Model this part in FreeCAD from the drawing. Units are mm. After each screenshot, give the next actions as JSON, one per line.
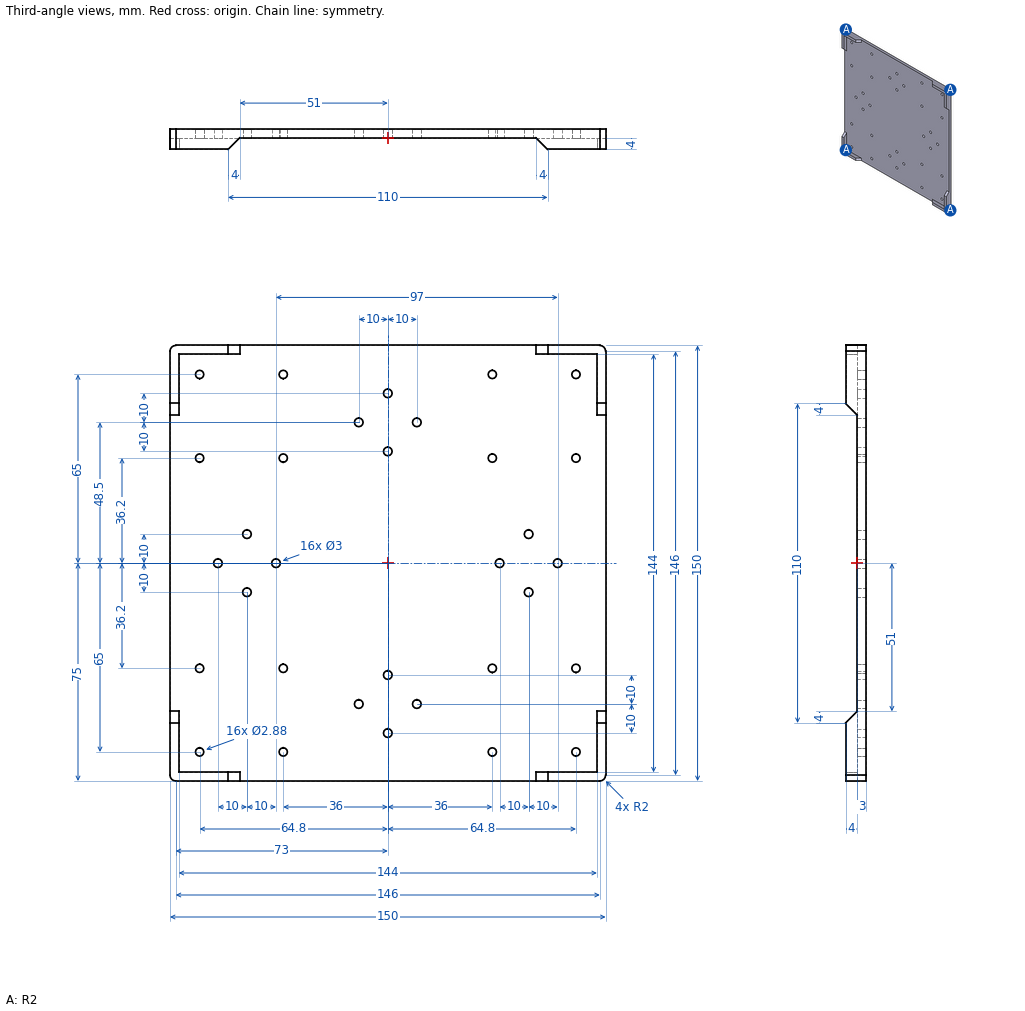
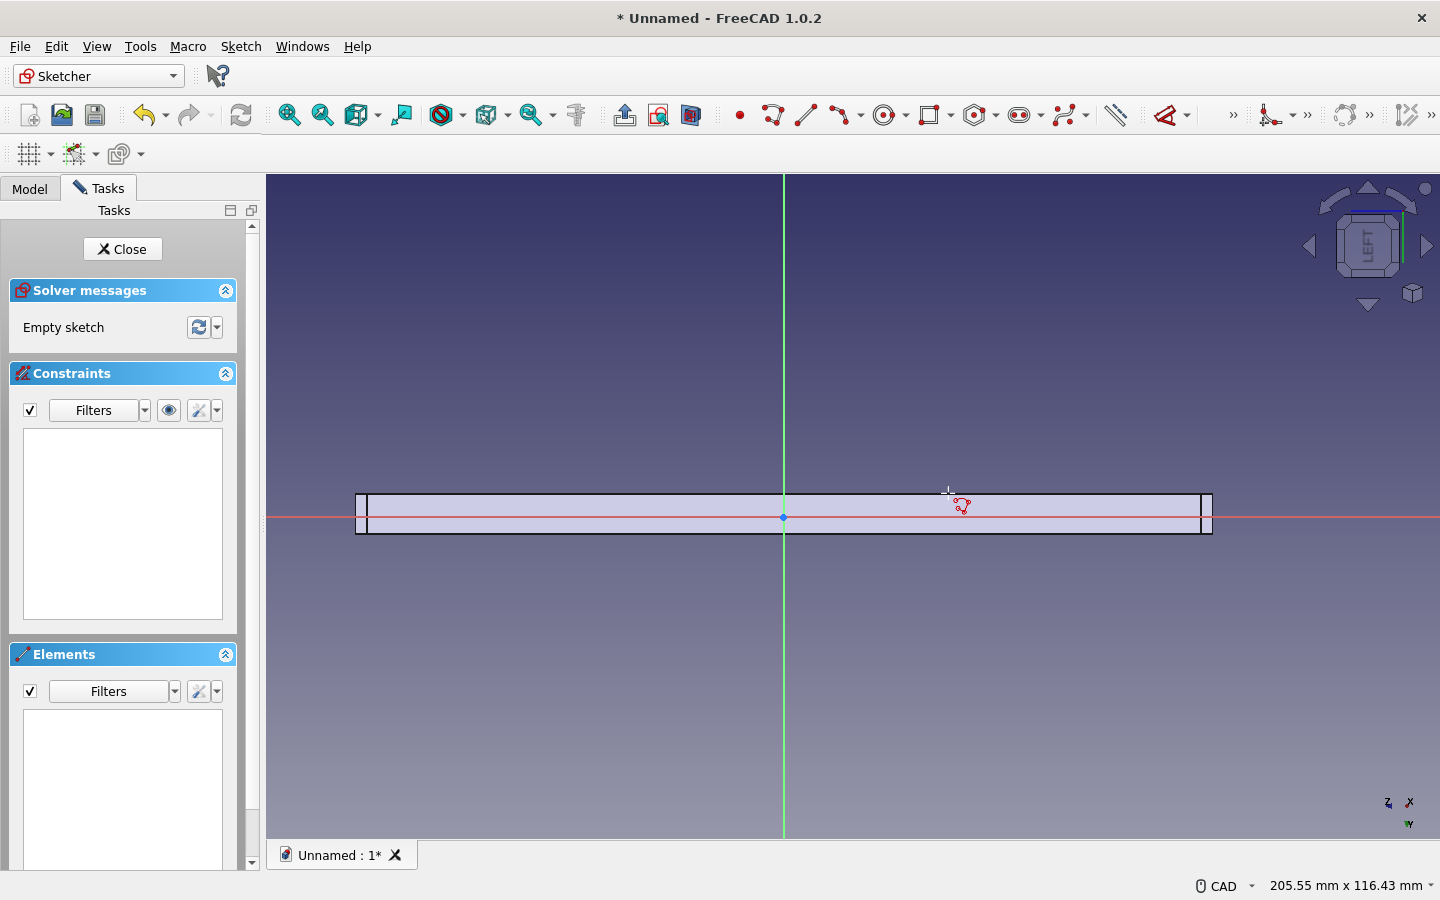
{"action": "left_click", "coordinate": [1075, 517]}
{"action": "left_click", "coordinate": [1098, 494]}
{"action": "left_click", "coordinate": [470, 494]}
{"action": "left_click", "coordinate": [493, 508]}
{"action": "left_click", "coordinate": [1075, 517]}
{"action": "key", "text": "Escape"}
{"action": "key", "text": "Escape"}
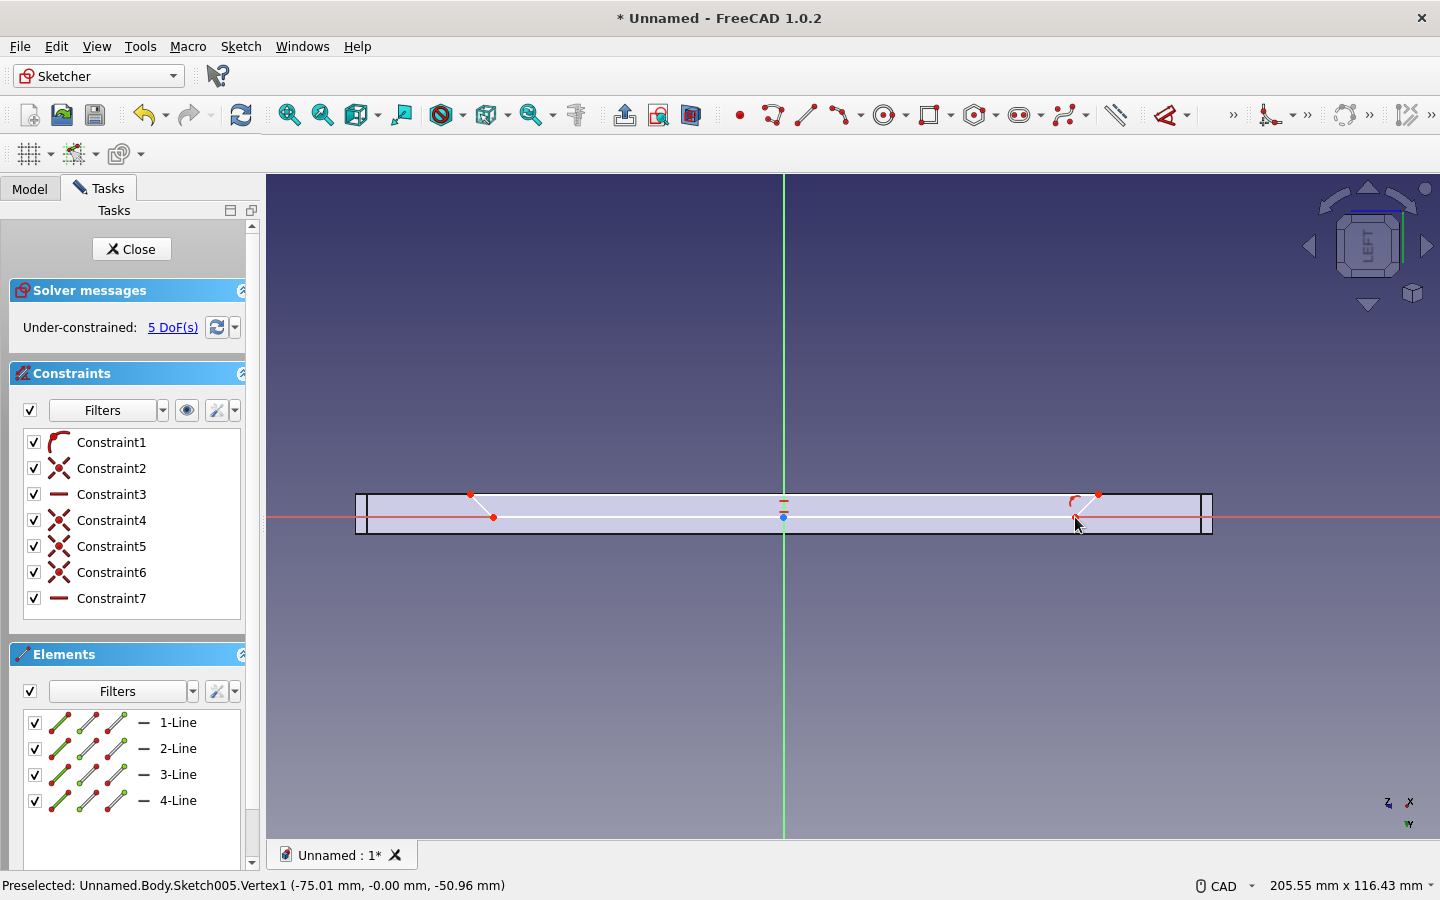
{"action": "key", "text": "d"}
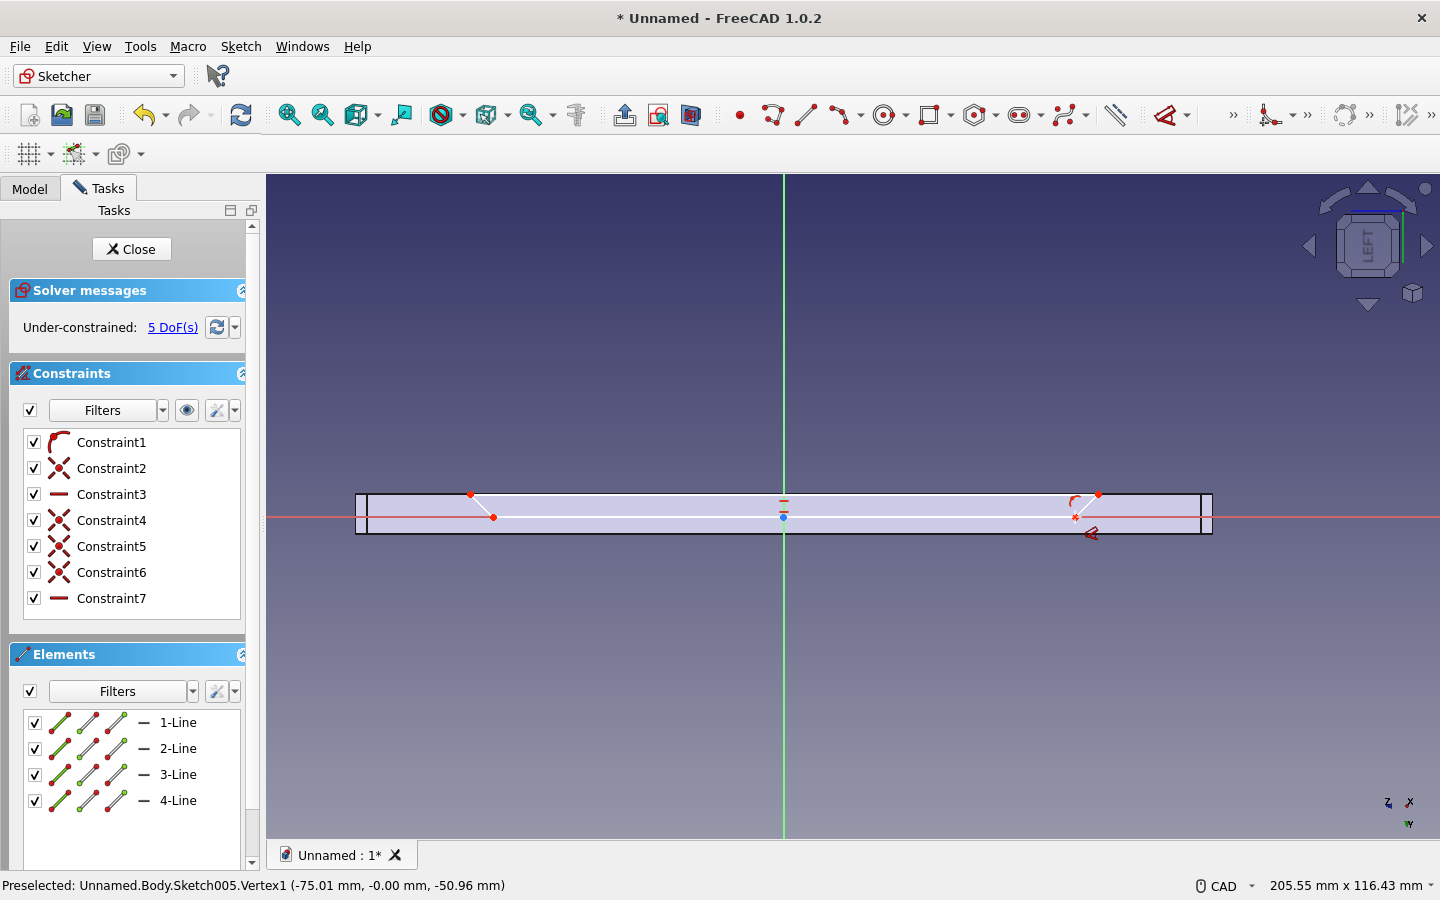
{"action": "scroll", "coordinate": [1098, 495], "scroll_direction": "up", "scroll_amount": 3}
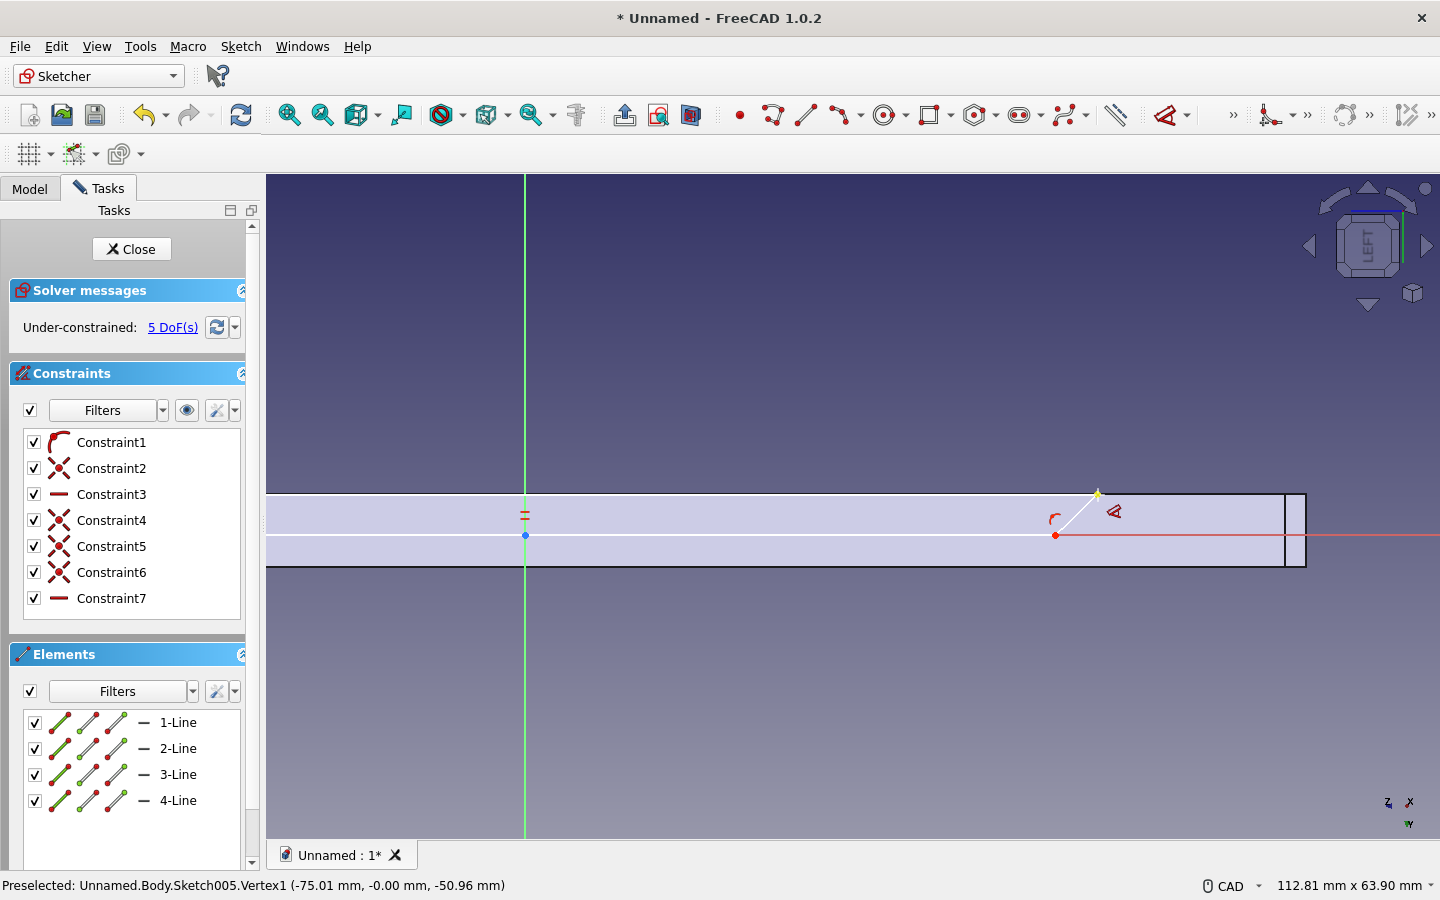
{"action": "left_click", "coordinate": [1097, 495]}
{"action": "left_click", "coordinate": [1131, 515]}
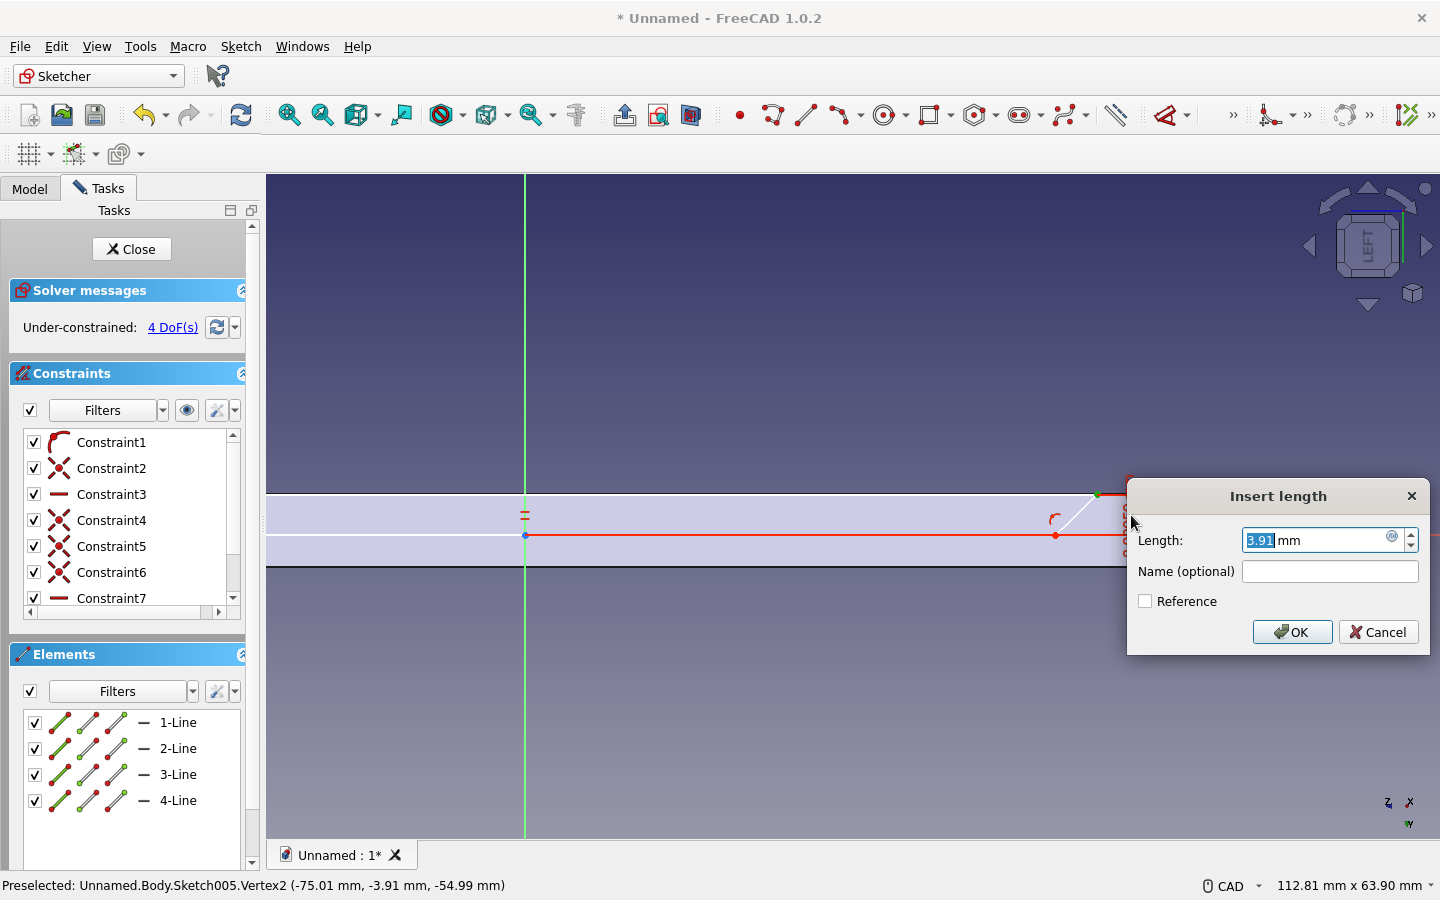
{"action": "type", "text": "4"}
{"action": "key", "text": "Return"}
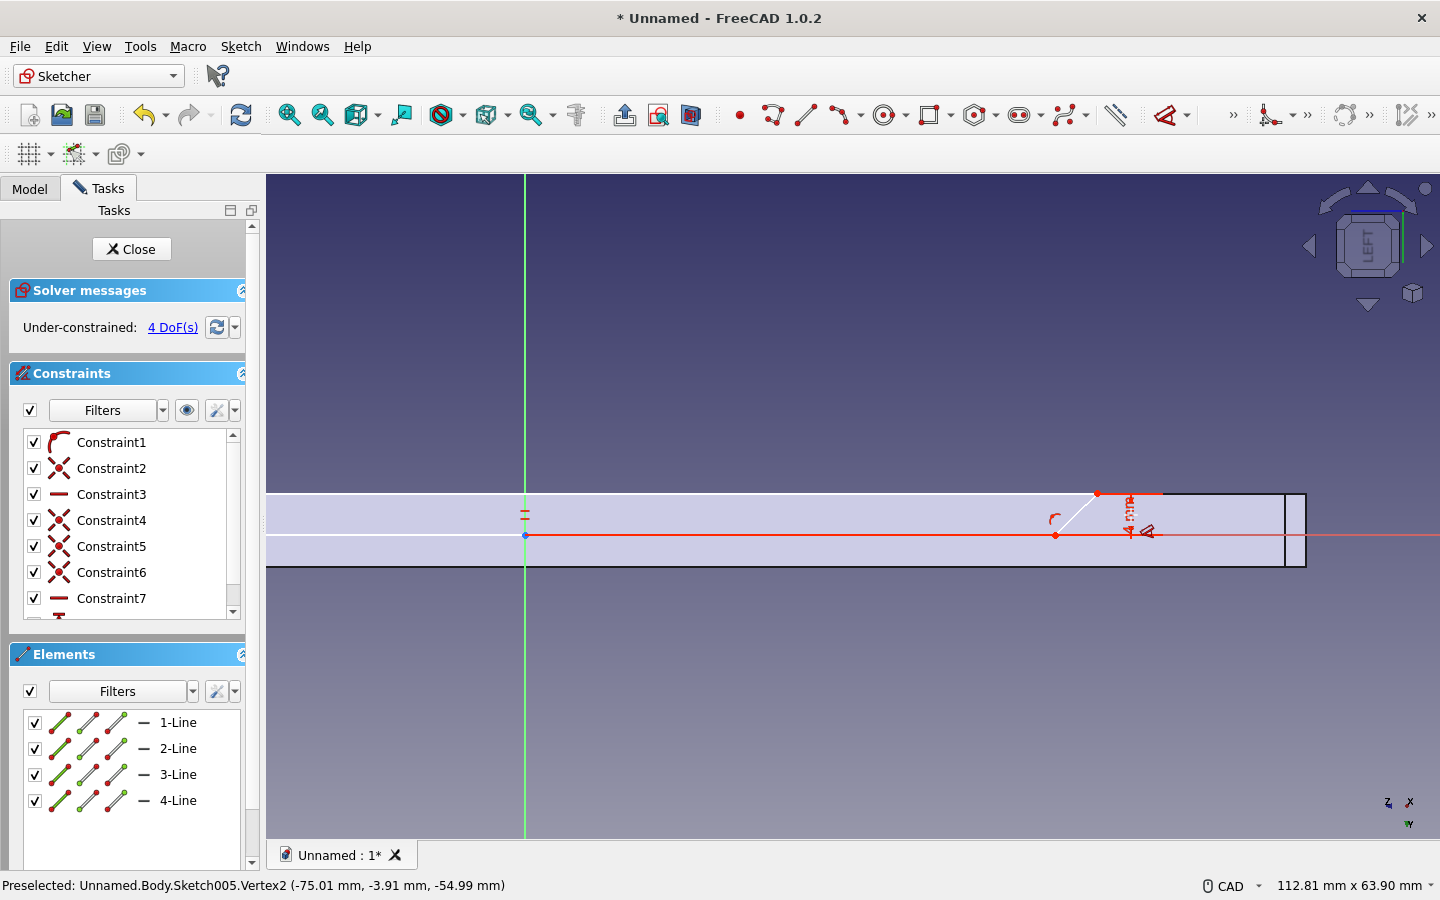
{"action": "left_click", "coordinate": [1068, 523]}
{"action": "left_click", "coordinate": [1076, 569]}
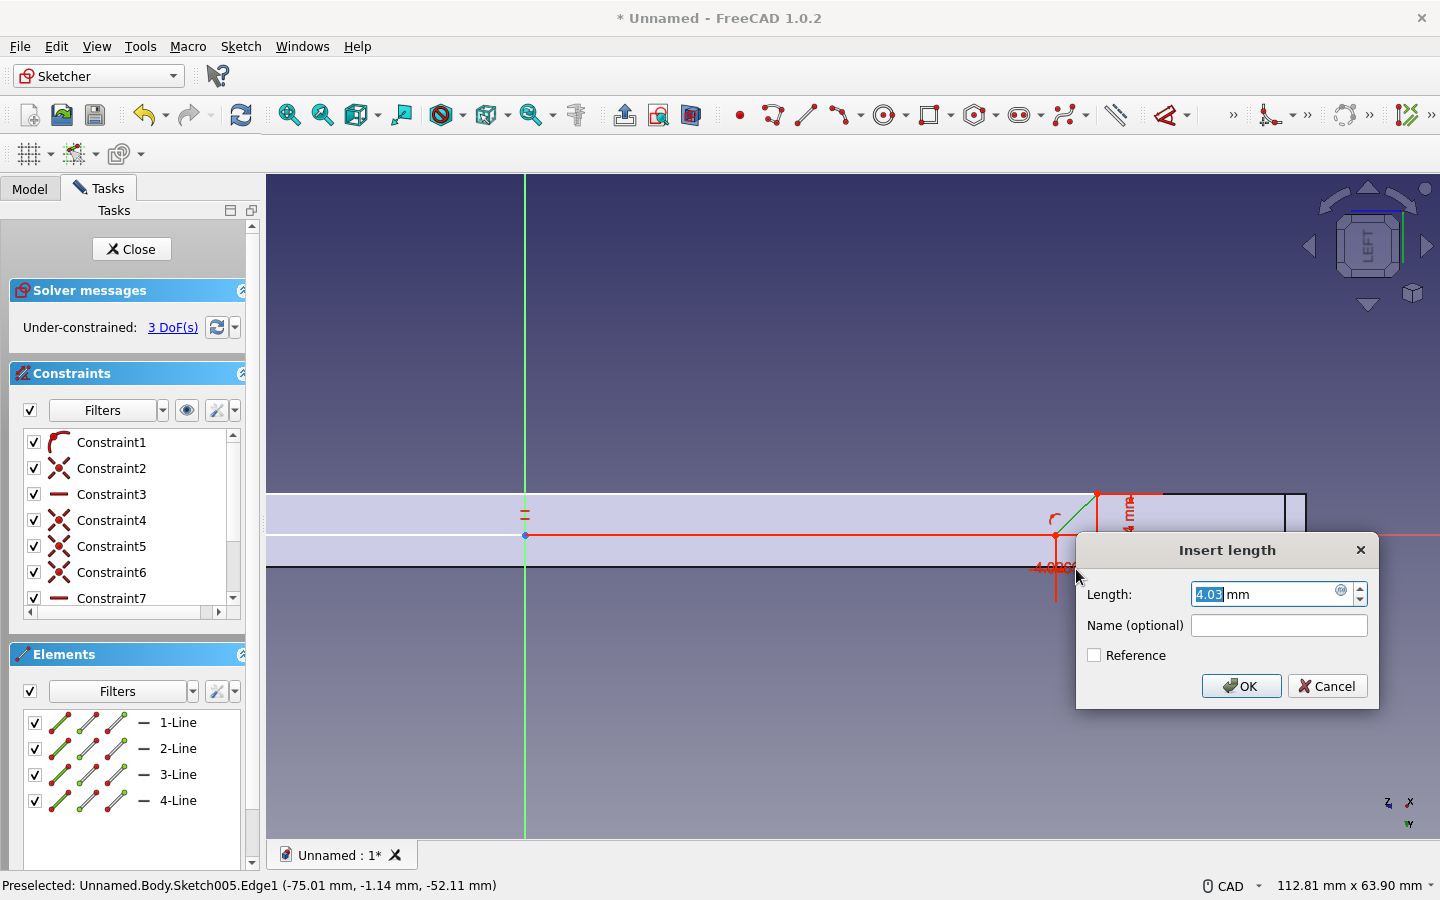
{"action": "type", "text": "4"}
{"action": "key", "text": "Return"}